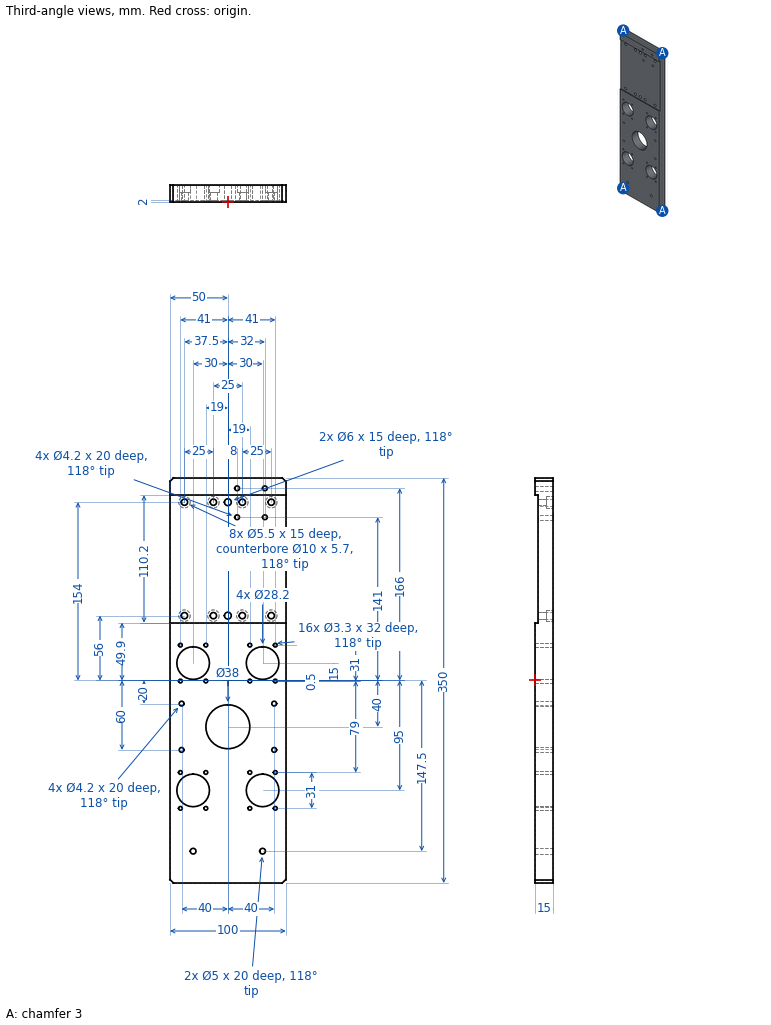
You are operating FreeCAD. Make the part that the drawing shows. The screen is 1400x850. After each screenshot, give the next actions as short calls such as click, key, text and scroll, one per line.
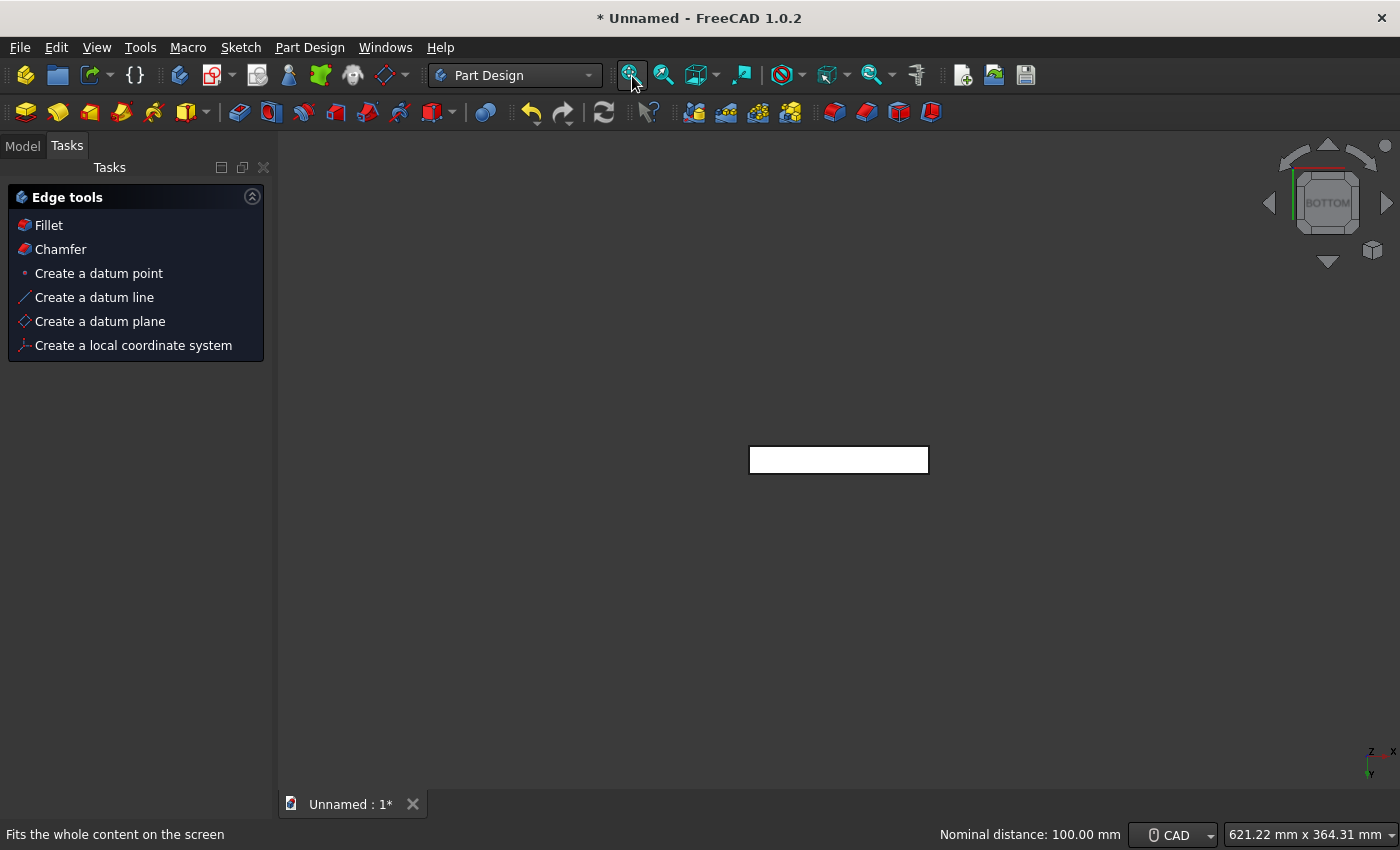
click(749, 459, ctrl)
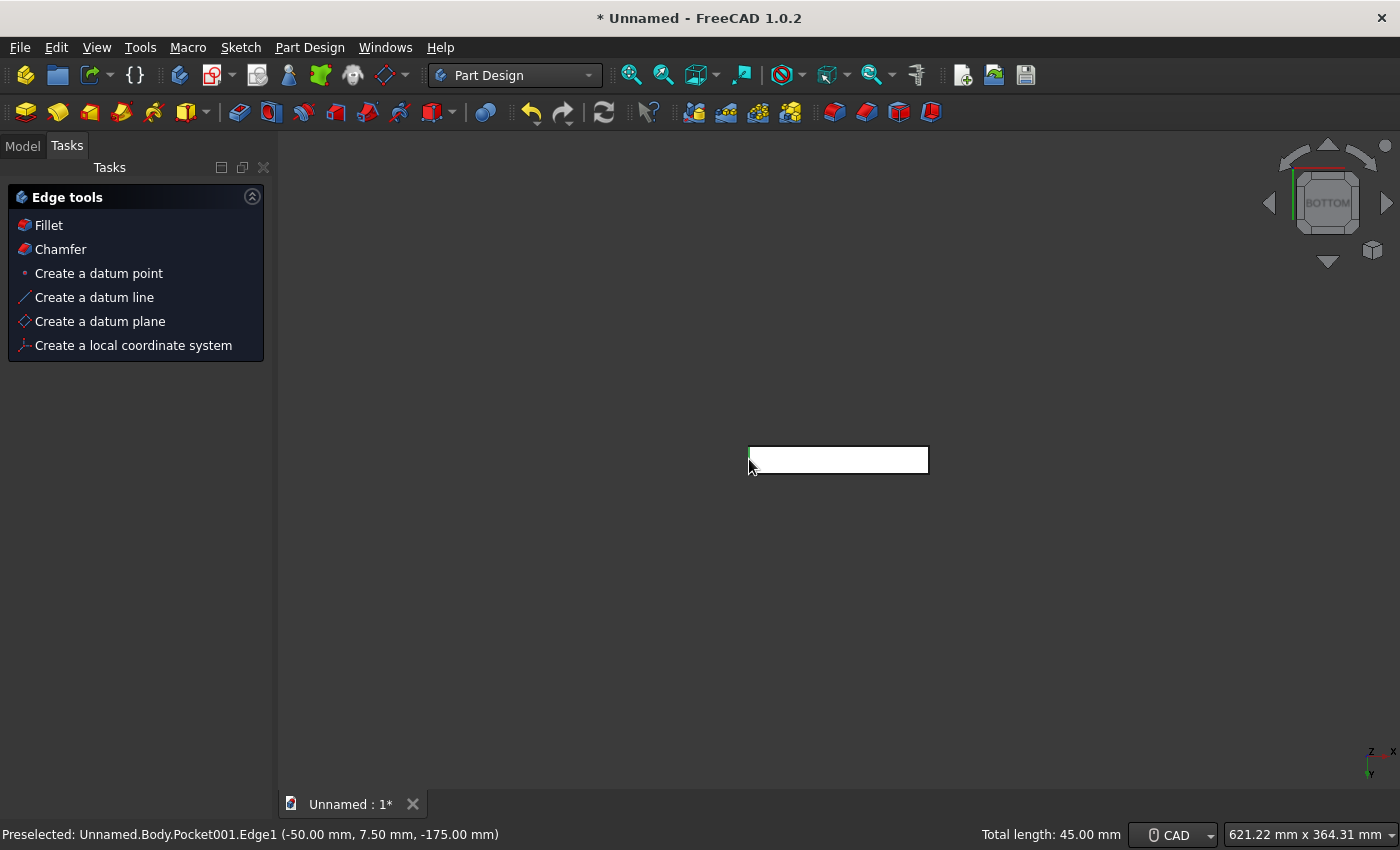
click(929, 459, ctrl)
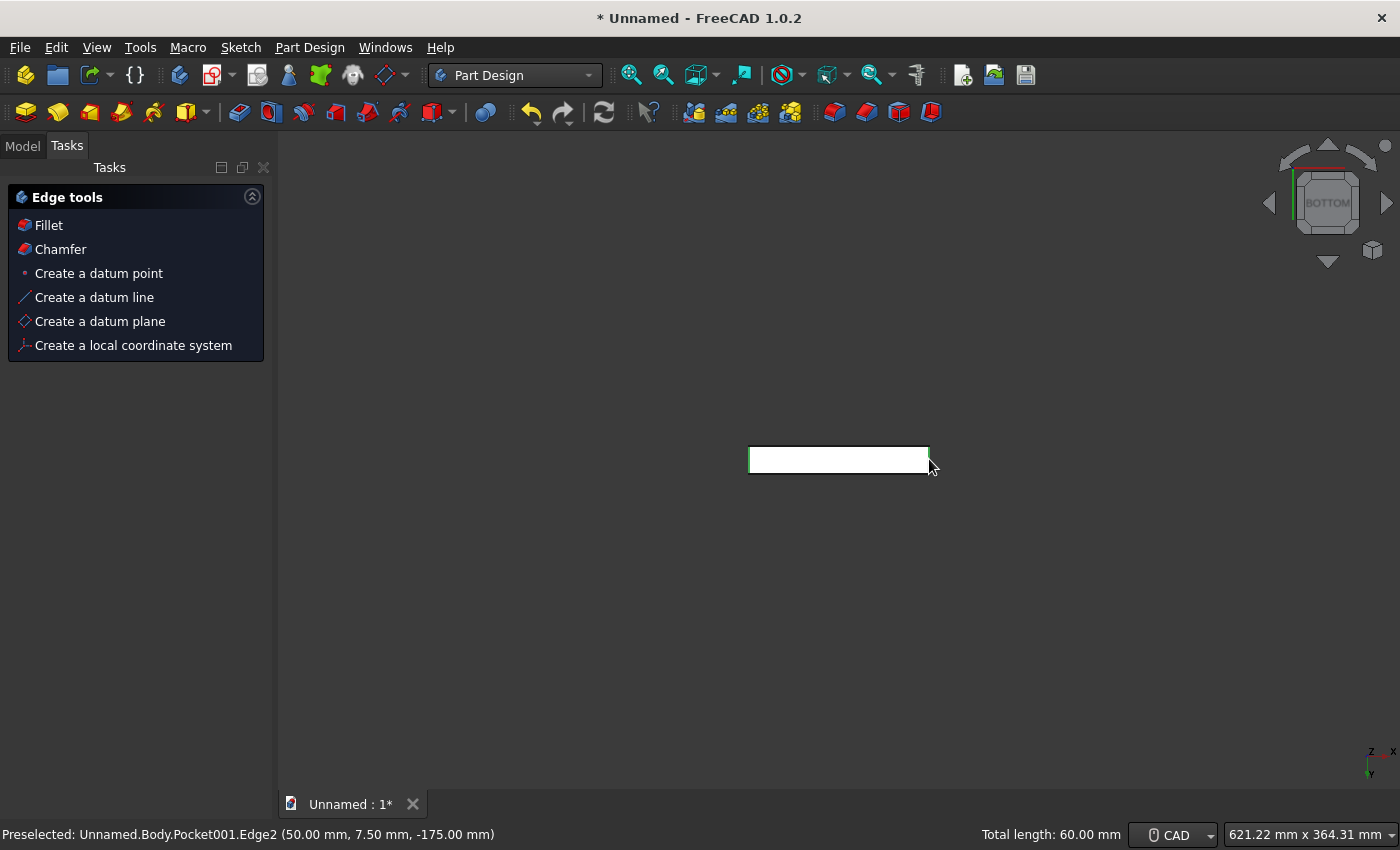
click(868, 112)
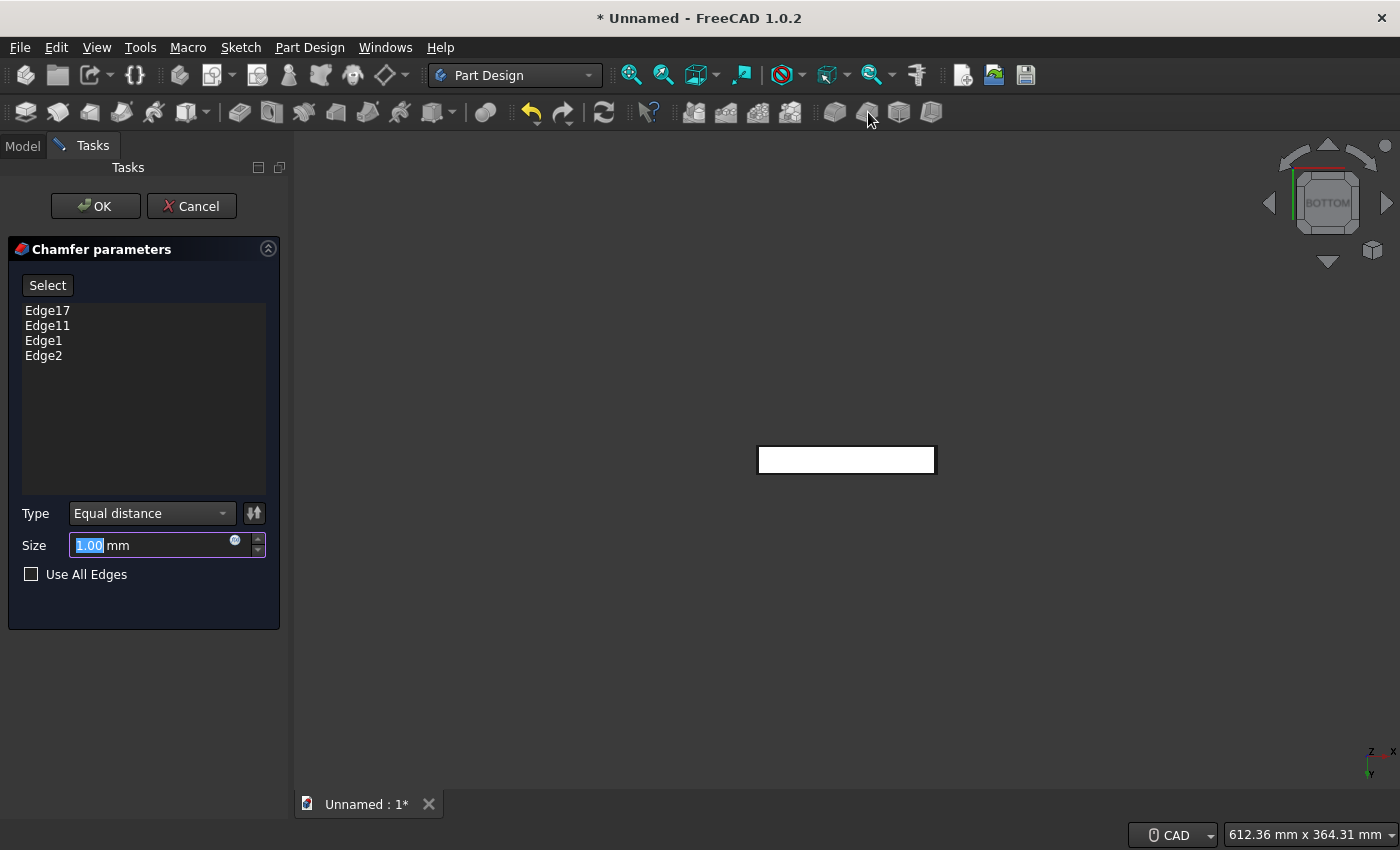
text(3)
key(Tab)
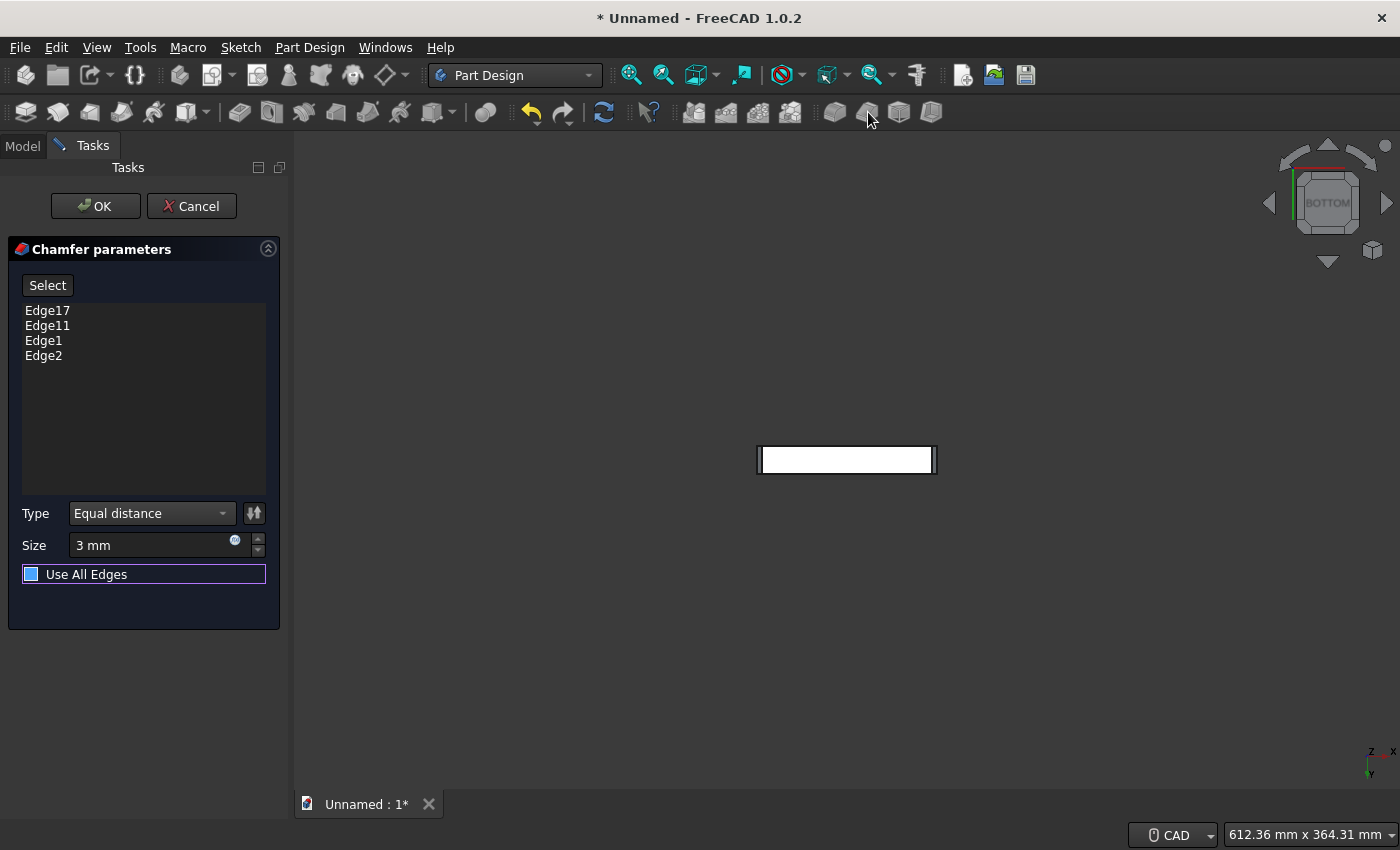
click(96, 206)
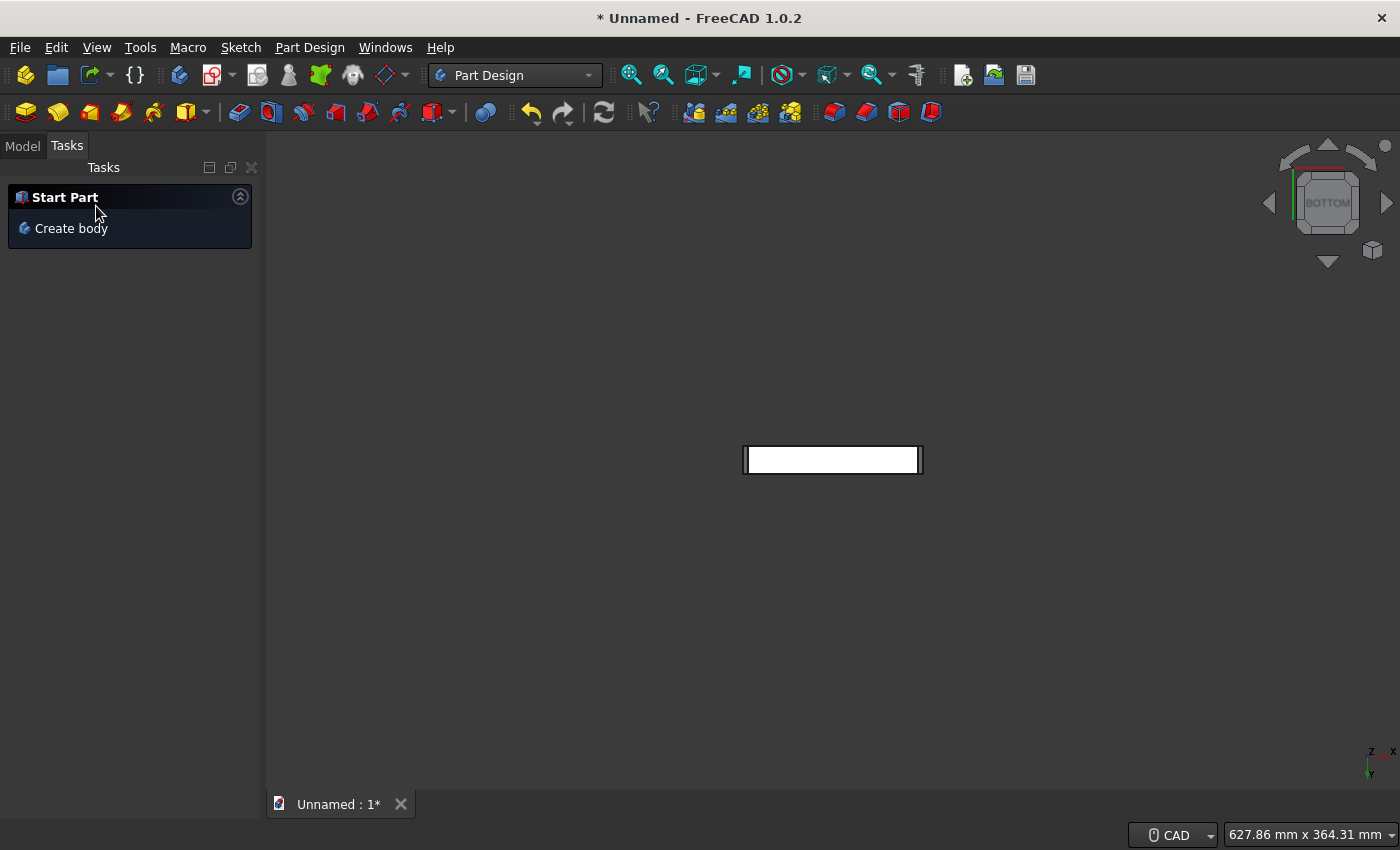
key(v)
key(f)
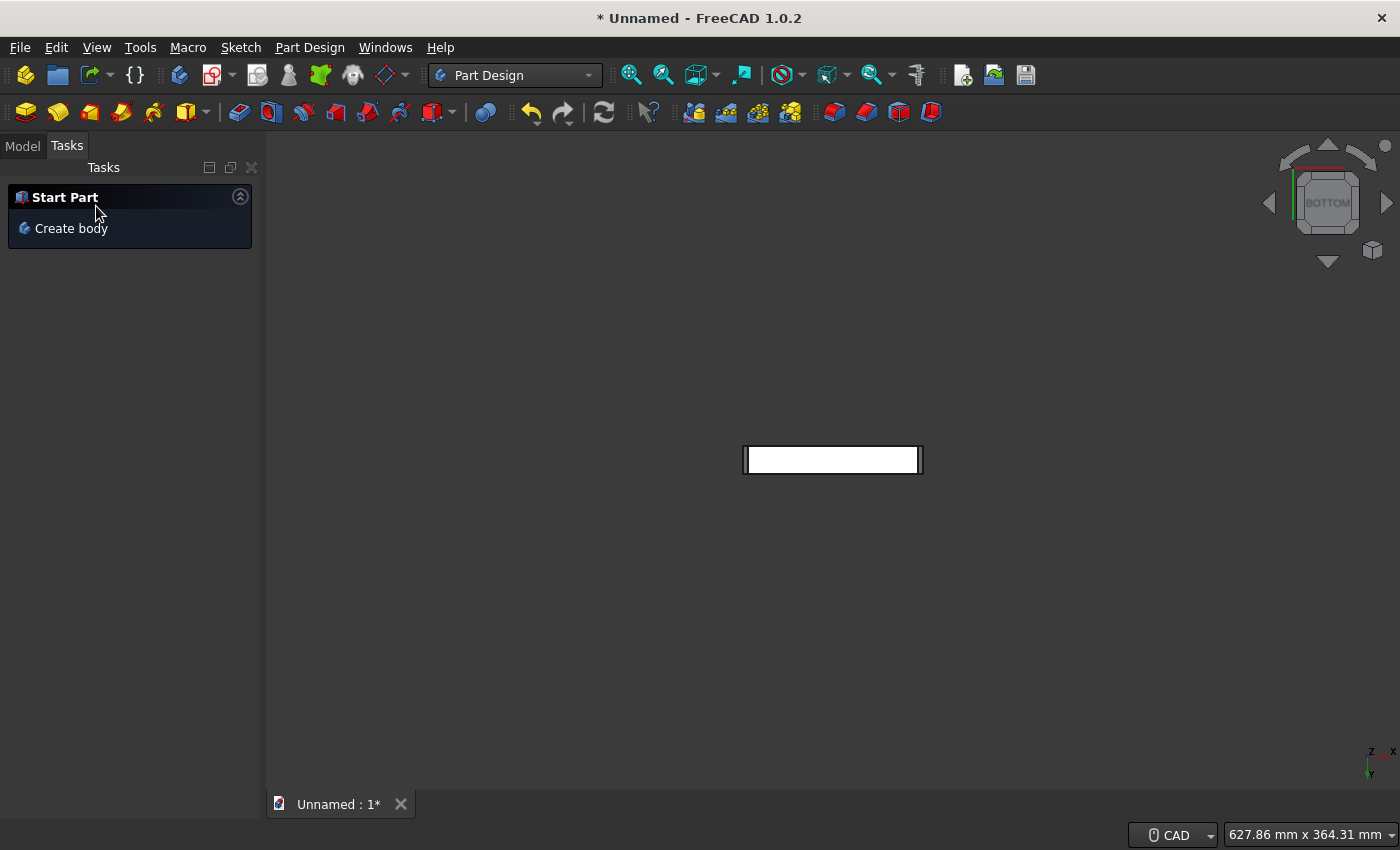
key(4)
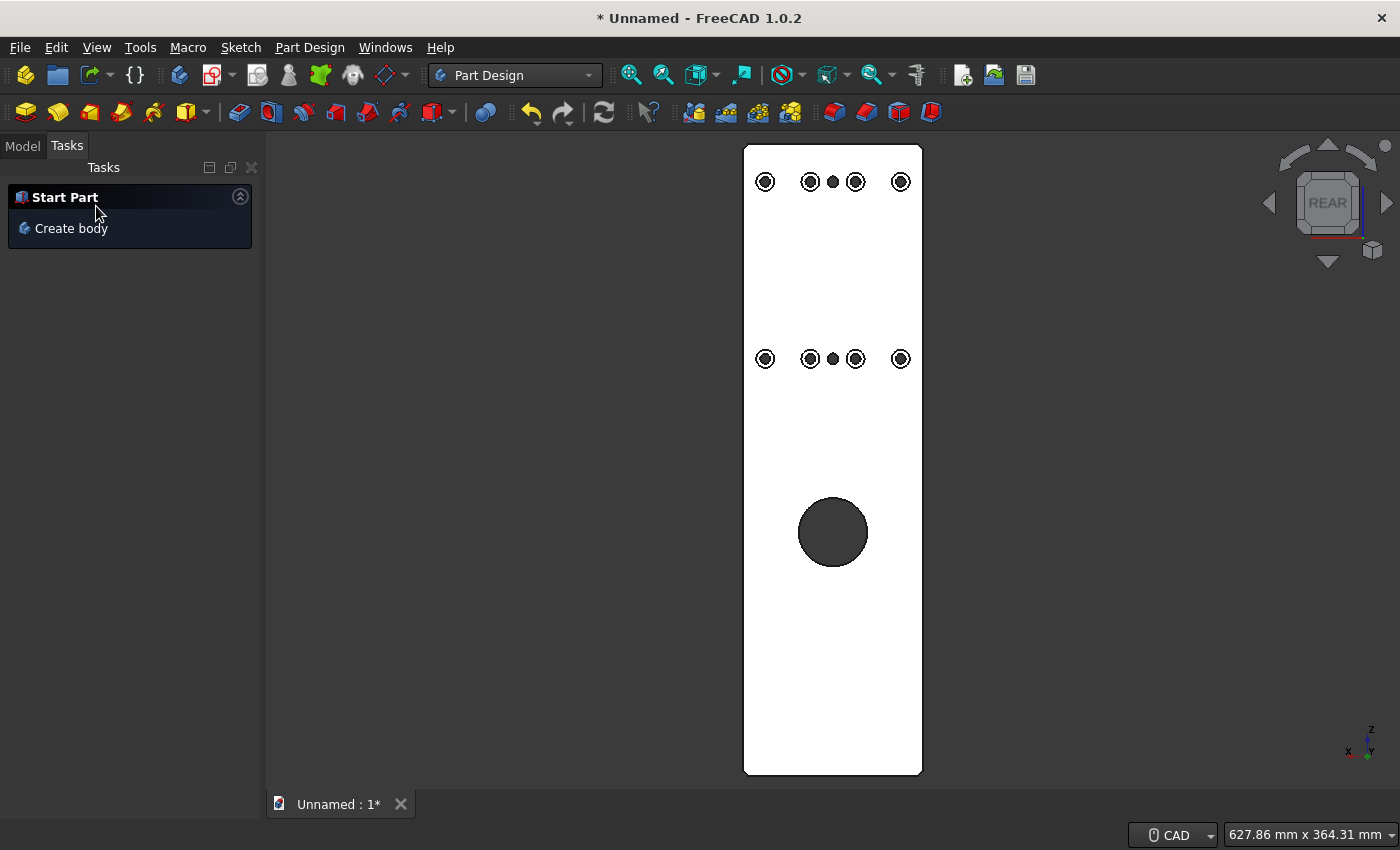
click(833, 640)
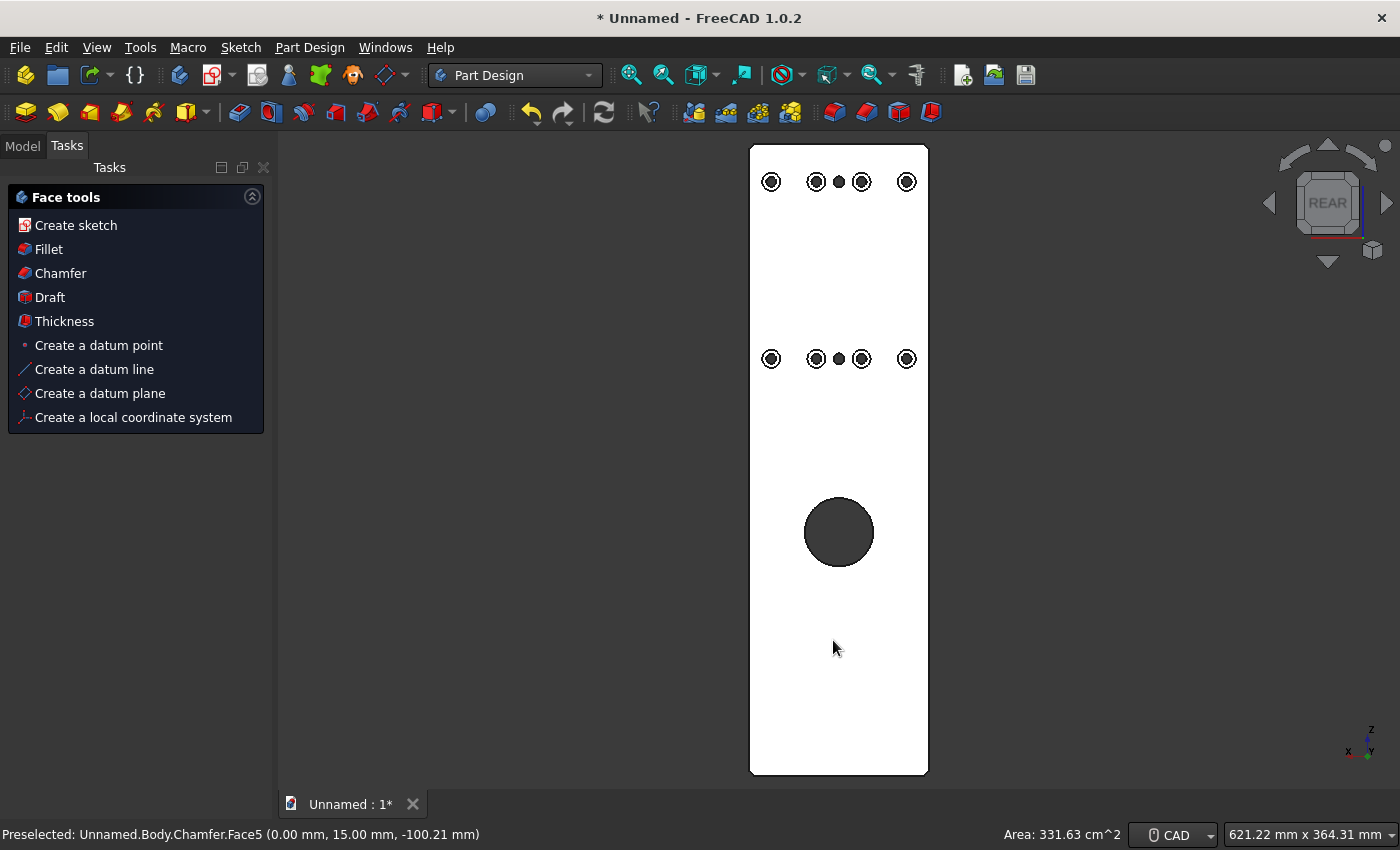
click(212, 76)